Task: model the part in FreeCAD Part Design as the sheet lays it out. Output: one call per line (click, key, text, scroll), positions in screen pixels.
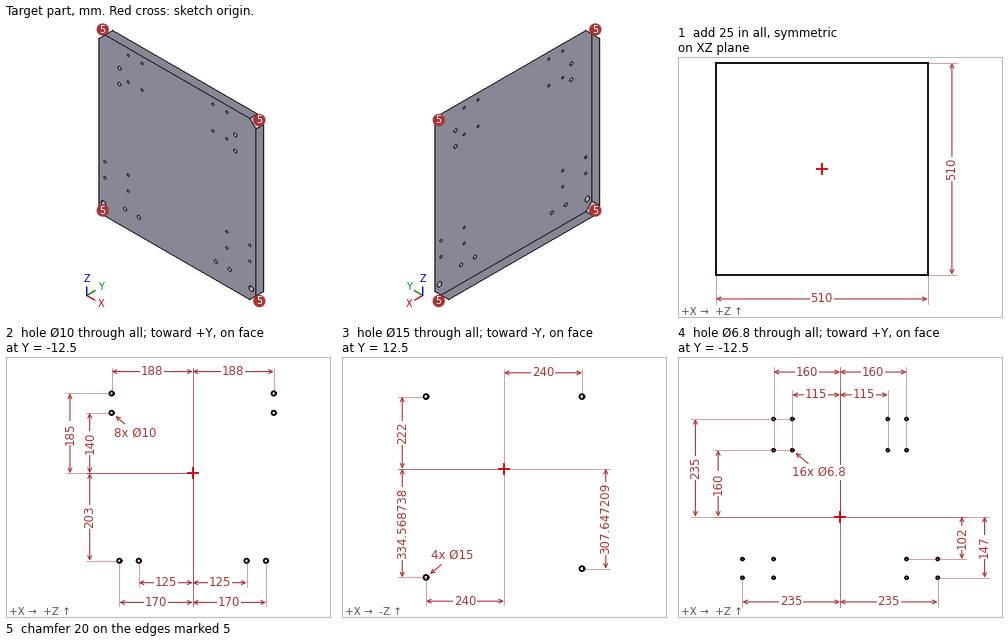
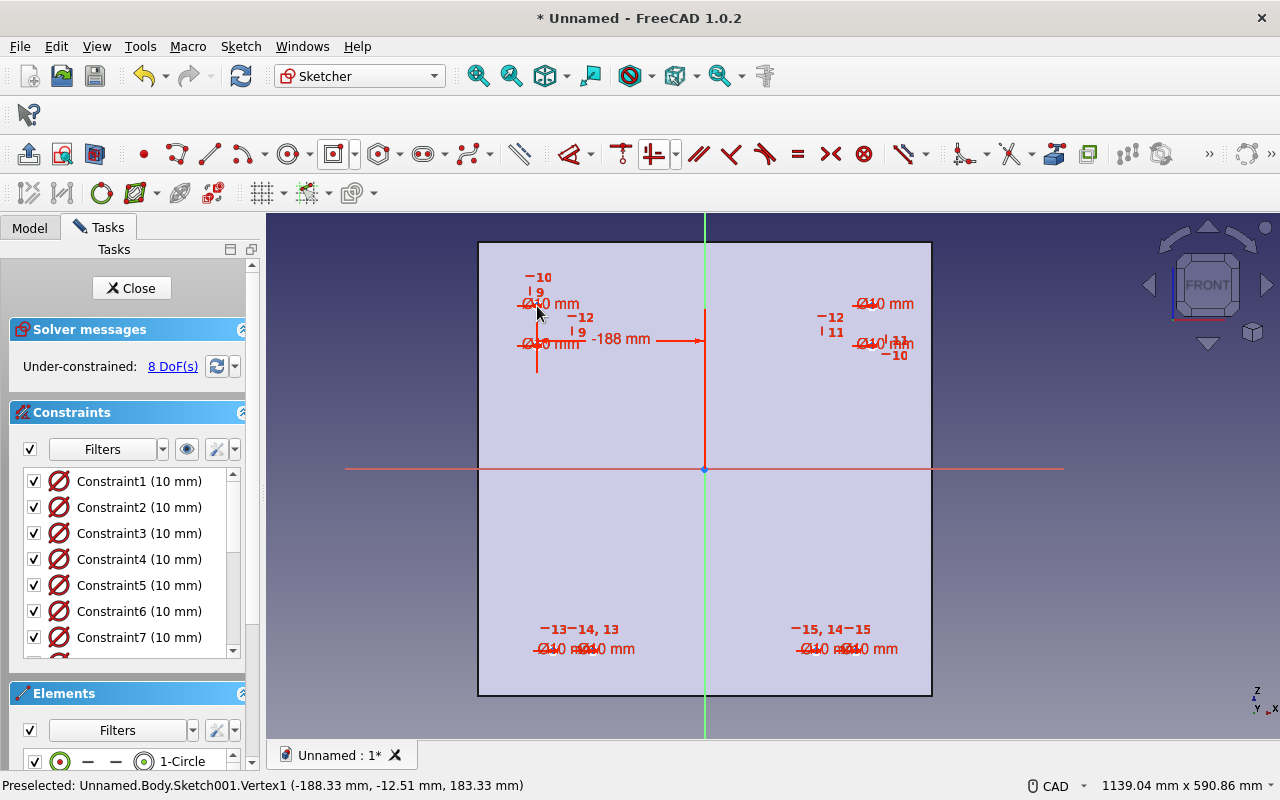
click(537, 306)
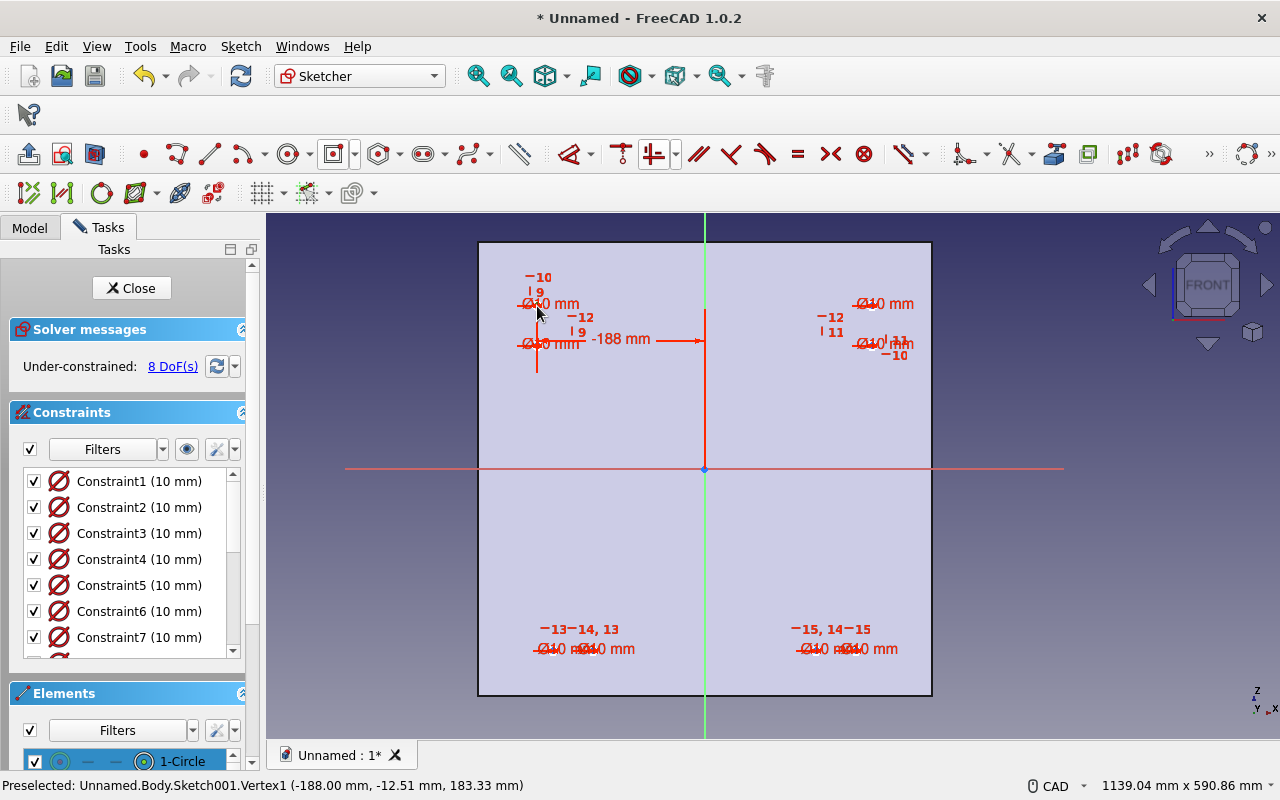
key(i)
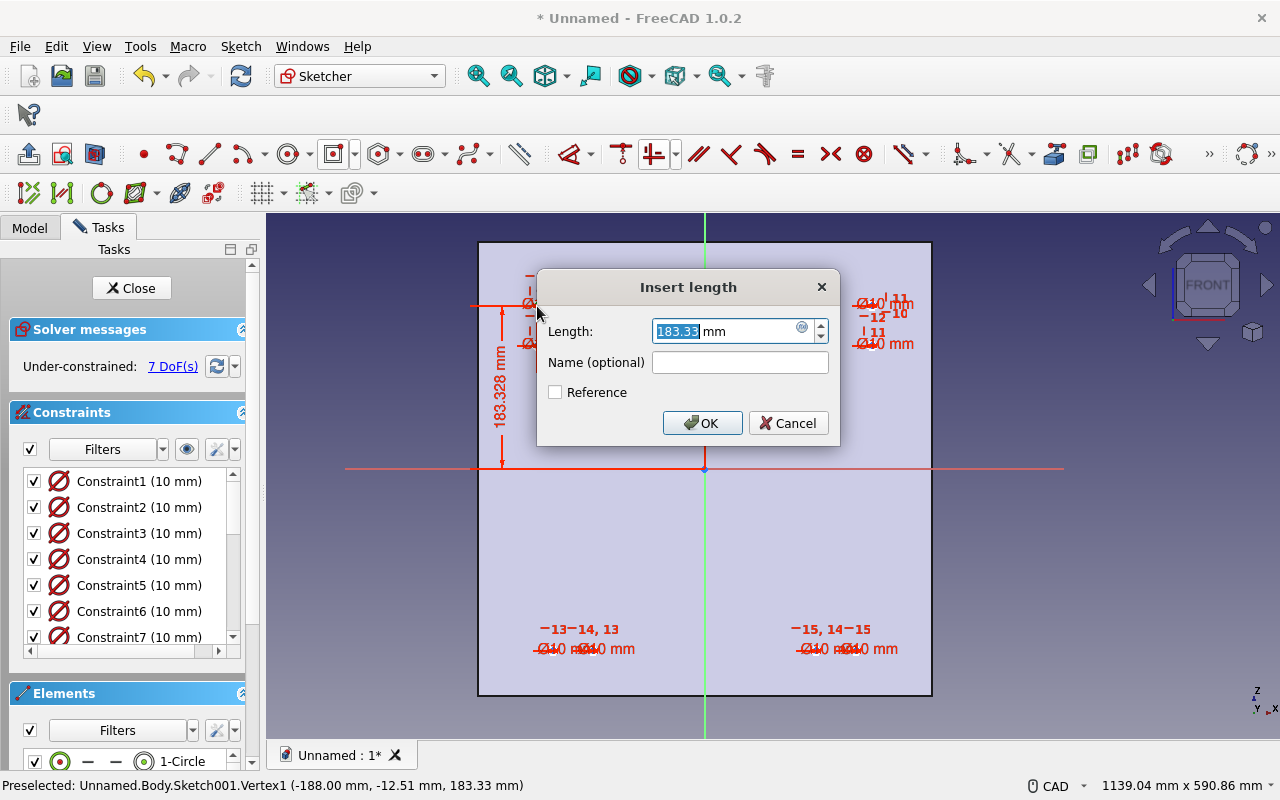
text(185)
key(Return)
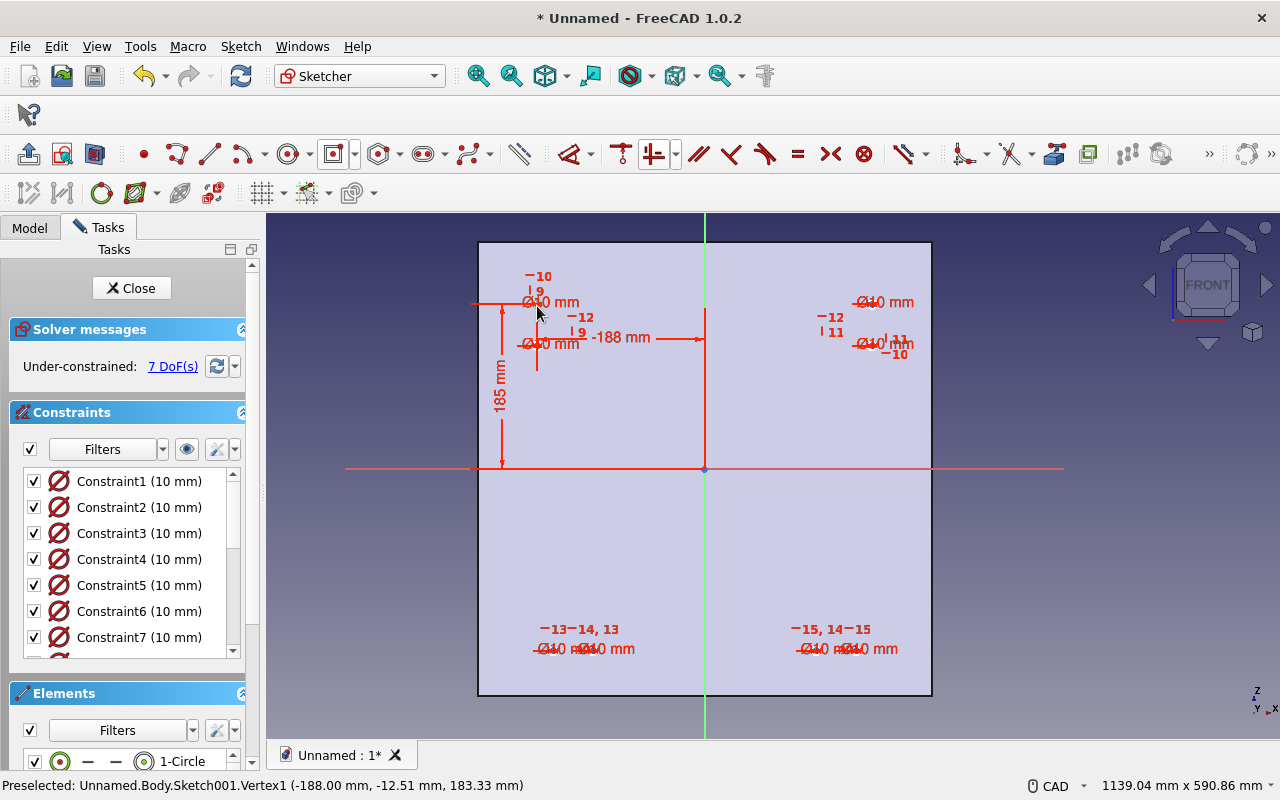
click(537, 346)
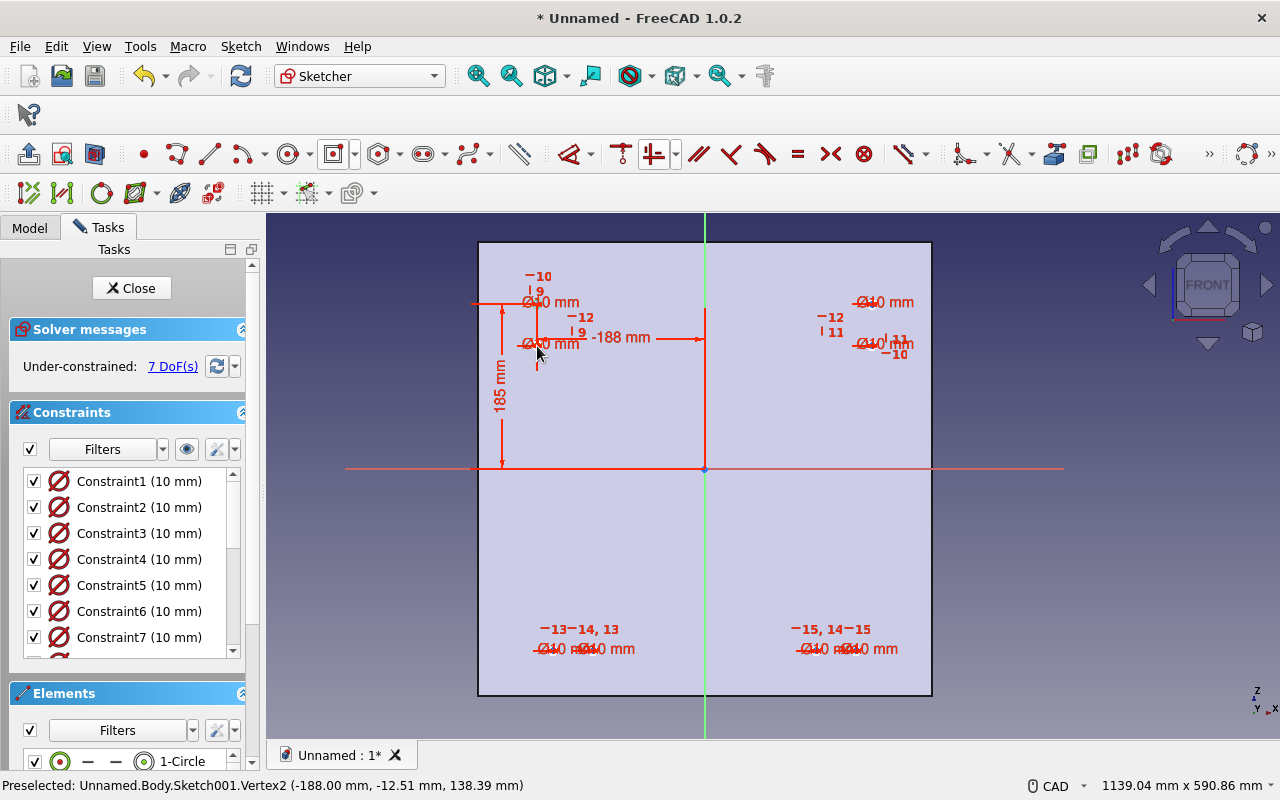
click(590, 154)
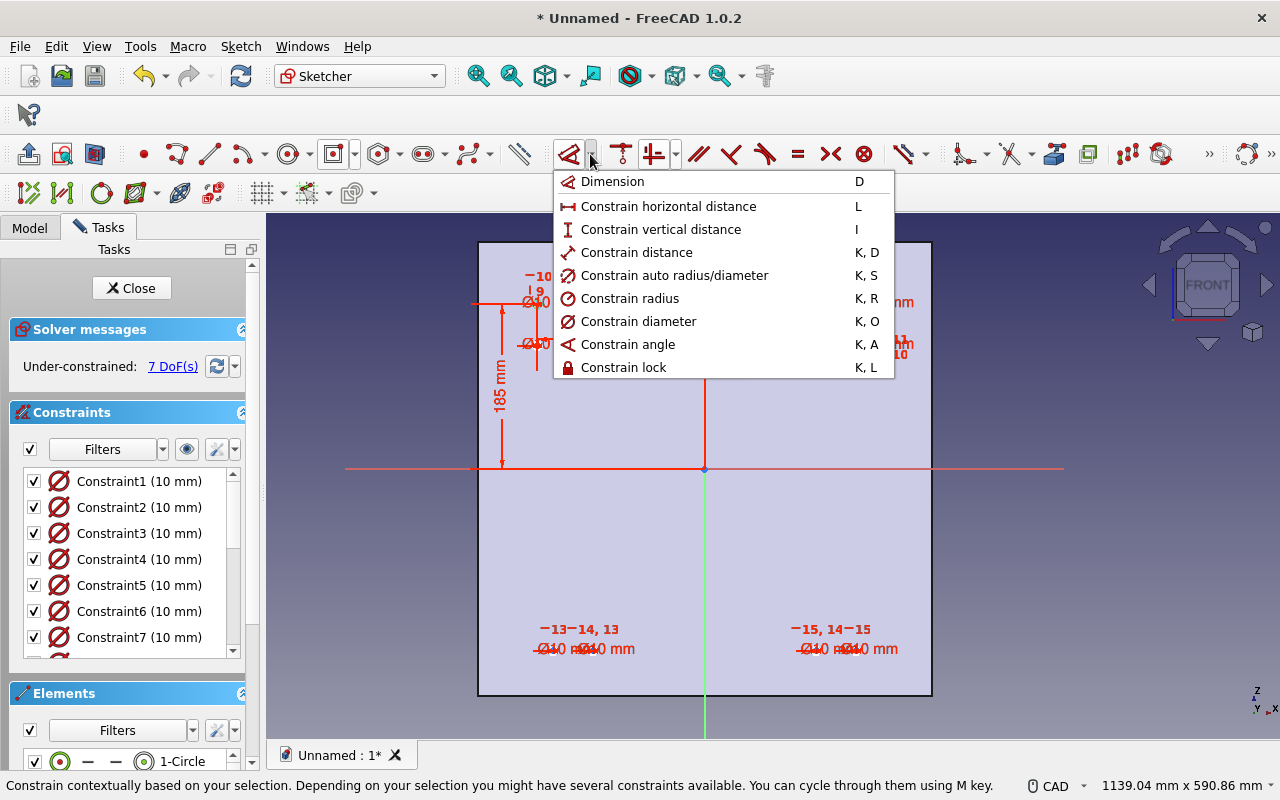
click(724, 230)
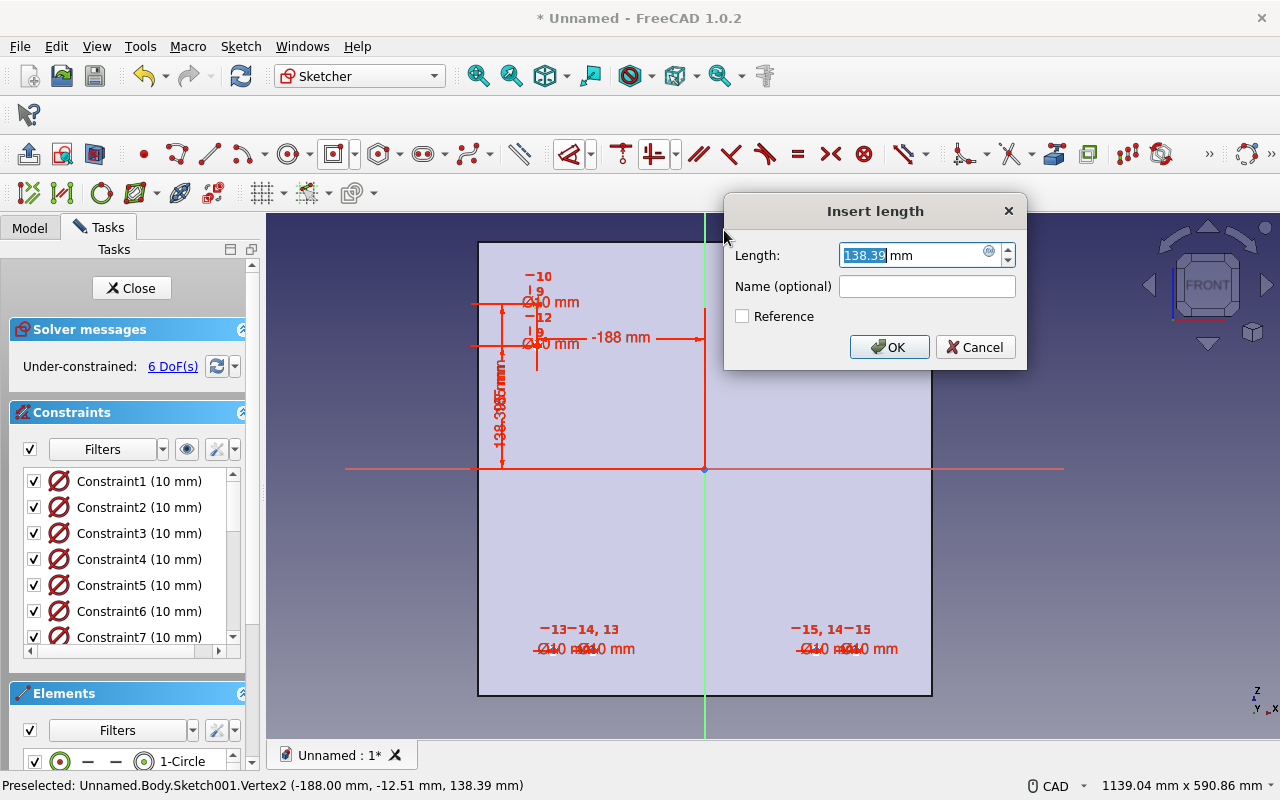
text(140)
key(Return)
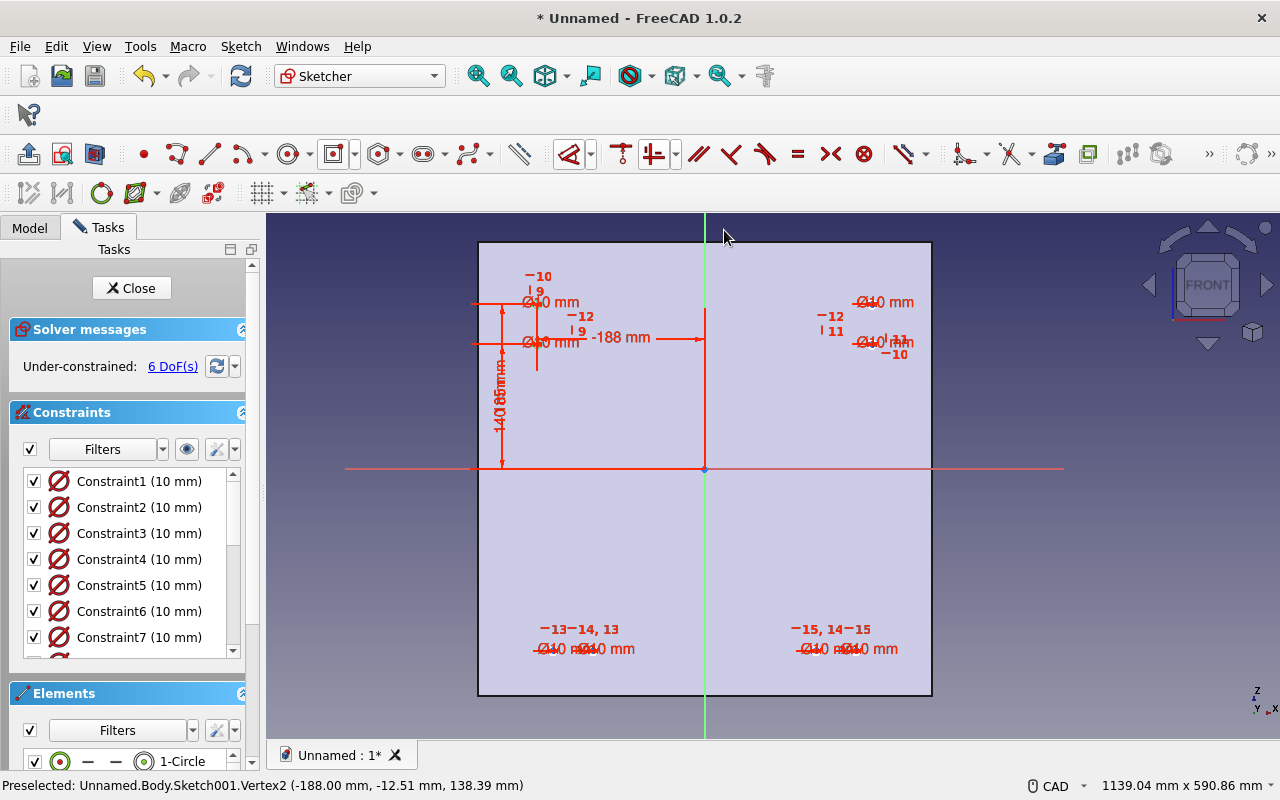
click(872, 304)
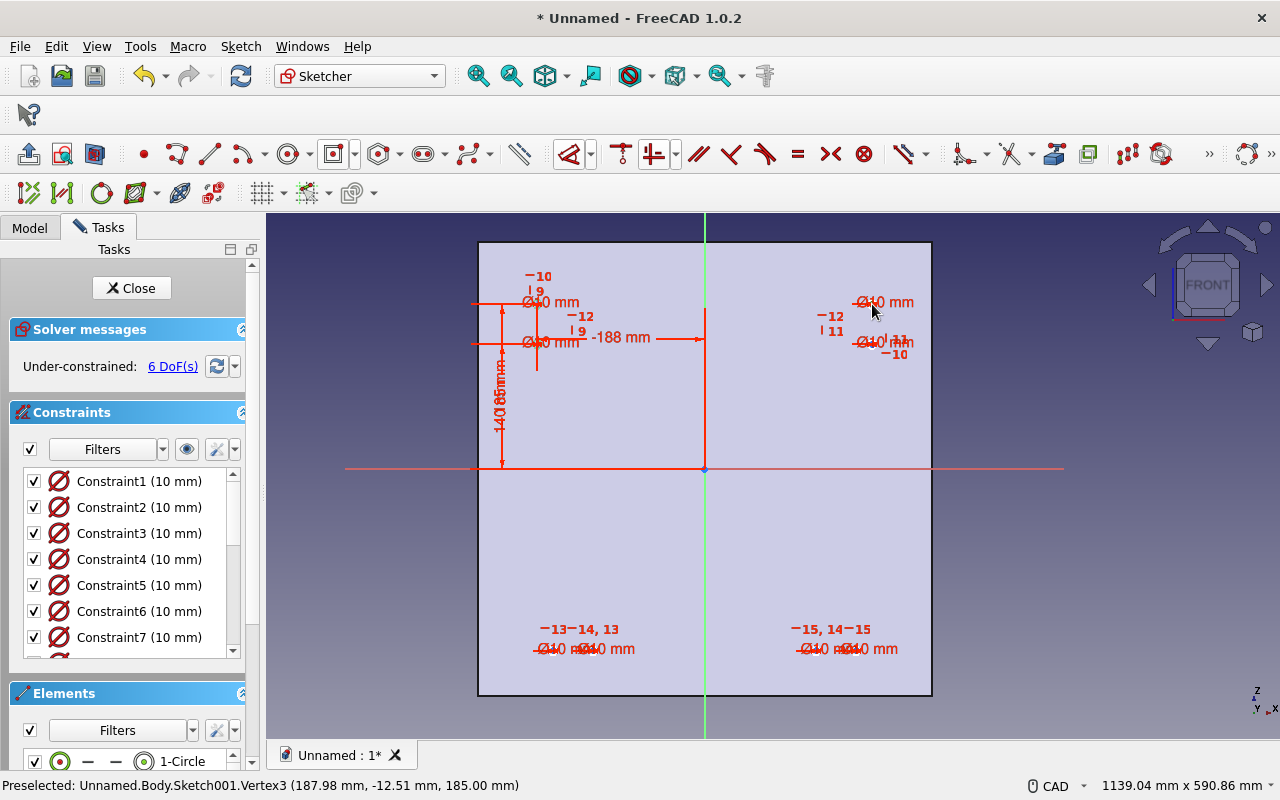
click(590, 154)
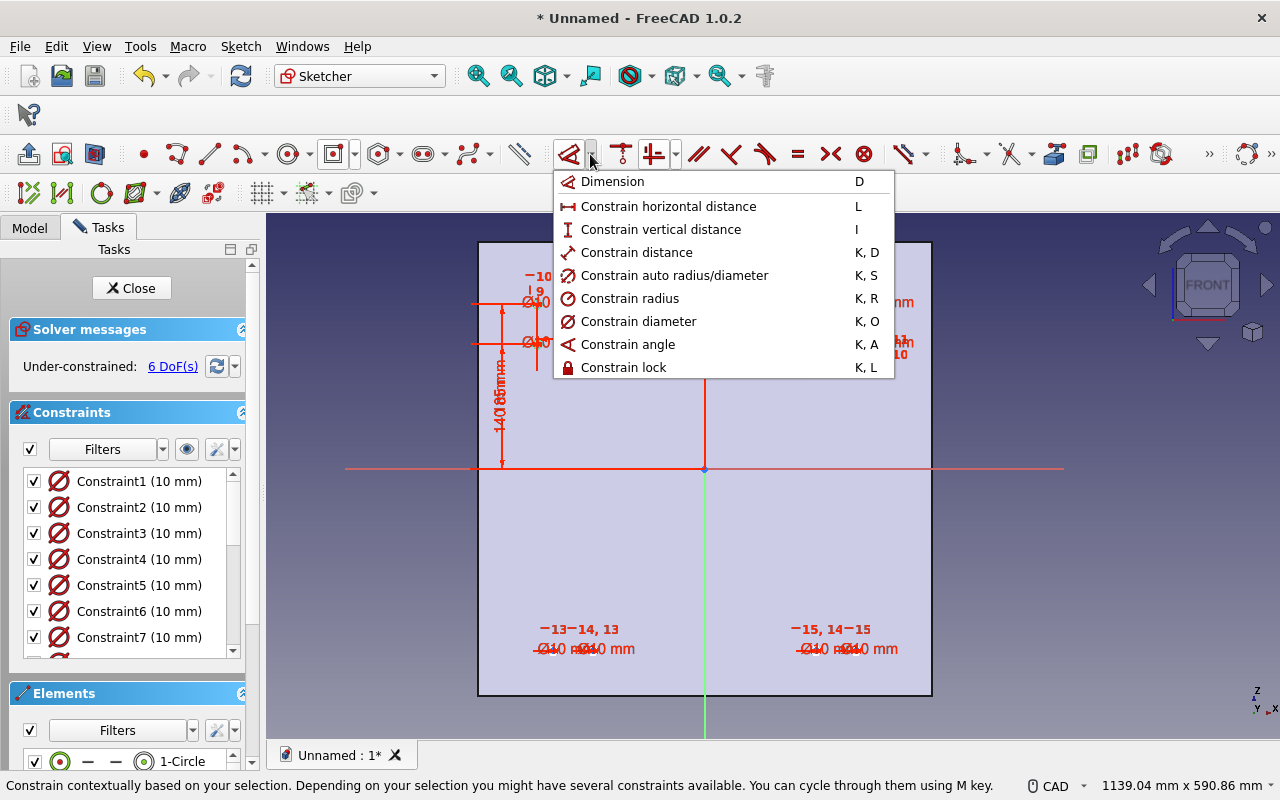
click(724, 206)